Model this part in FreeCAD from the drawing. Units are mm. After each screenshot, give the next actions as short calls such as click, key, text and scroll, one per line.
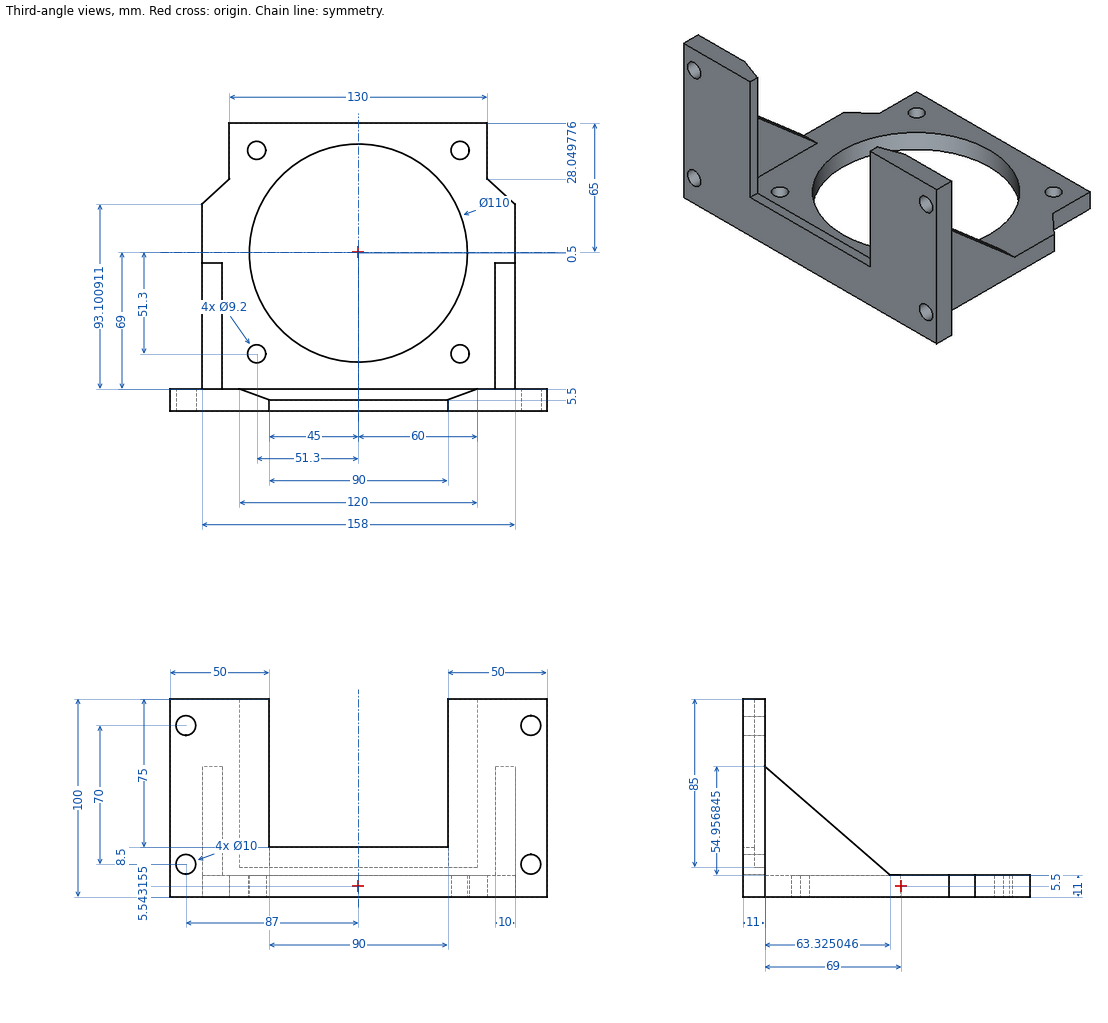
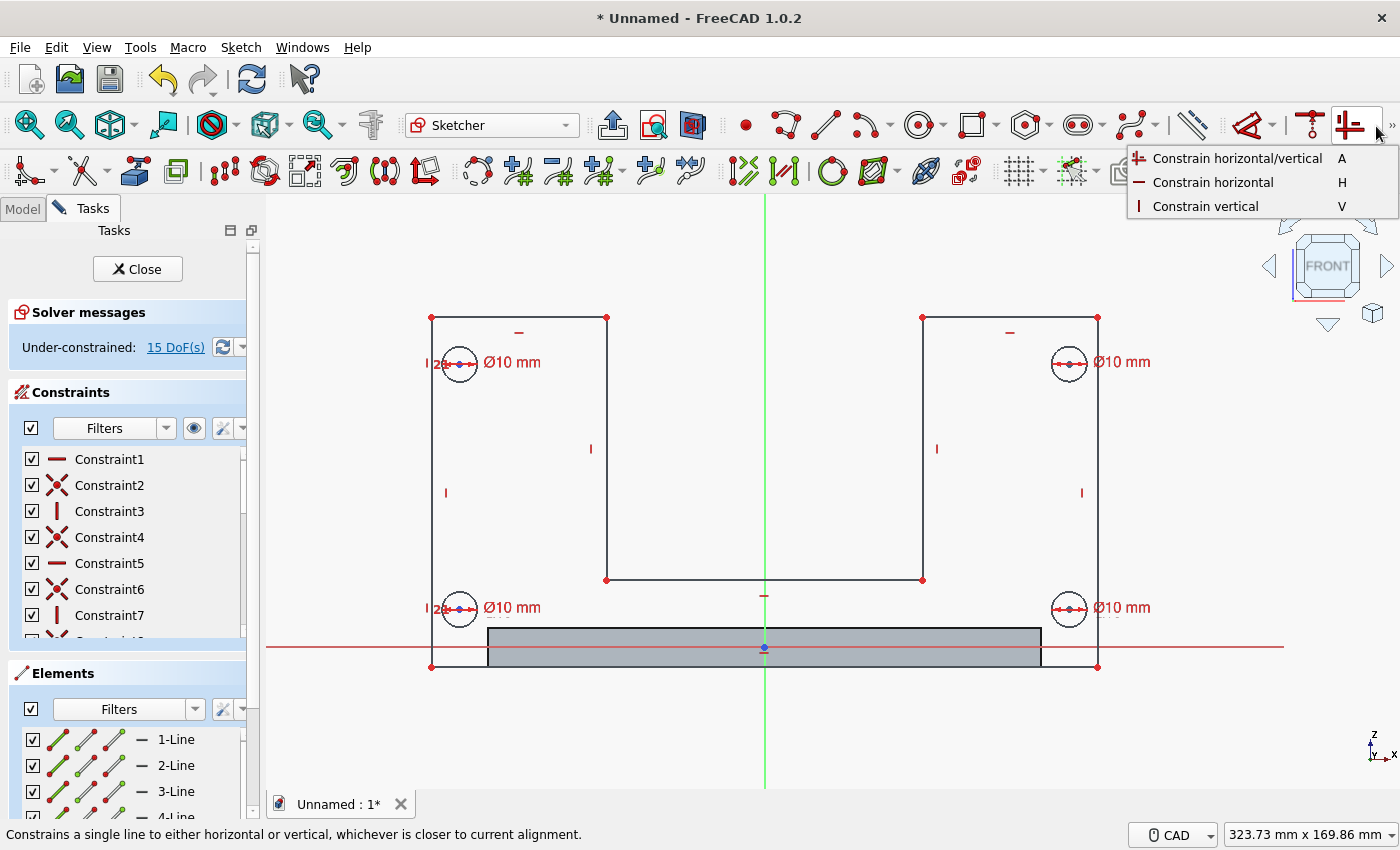
click(1263, 206)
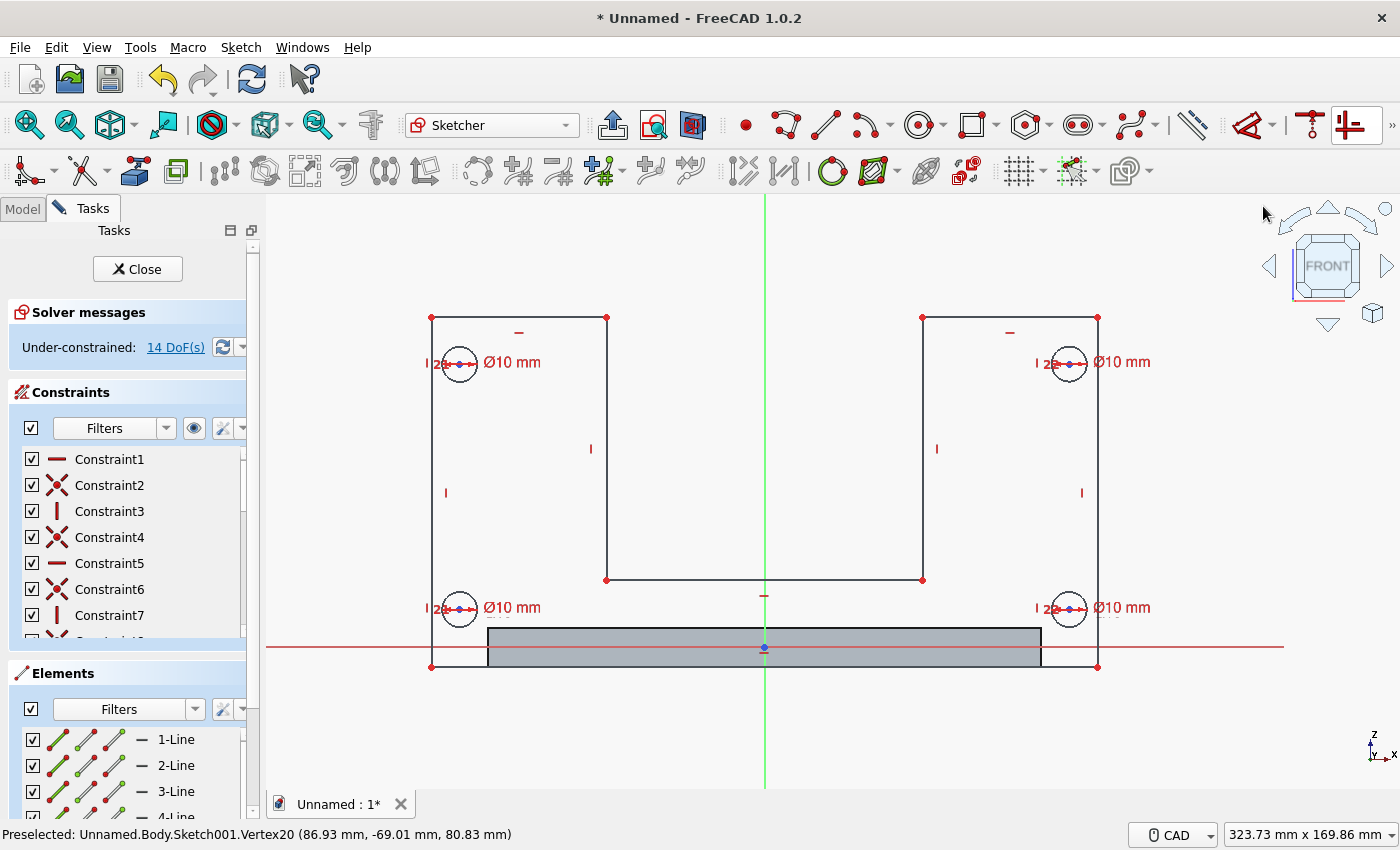
click(460, 610)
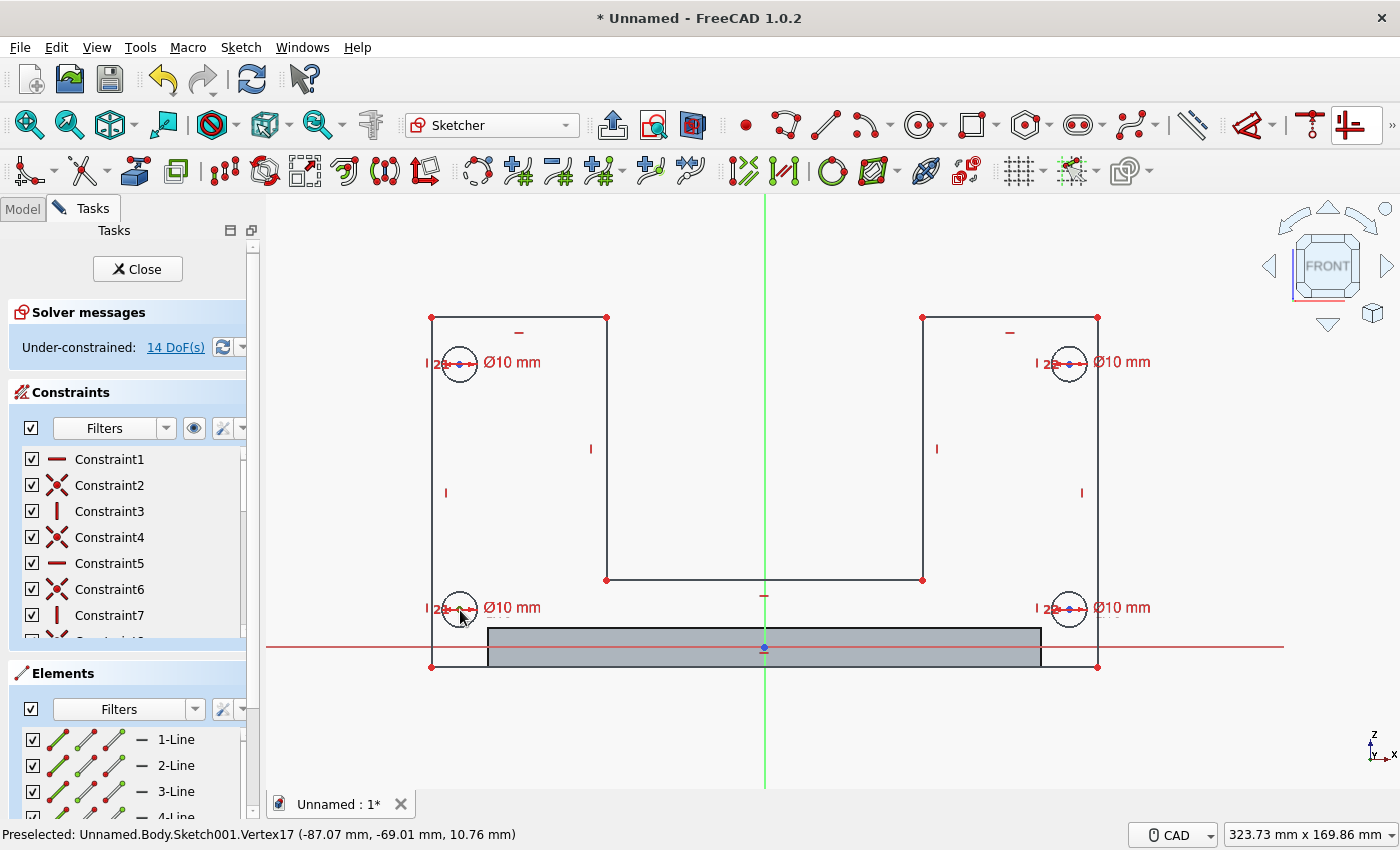
click(1069, 610)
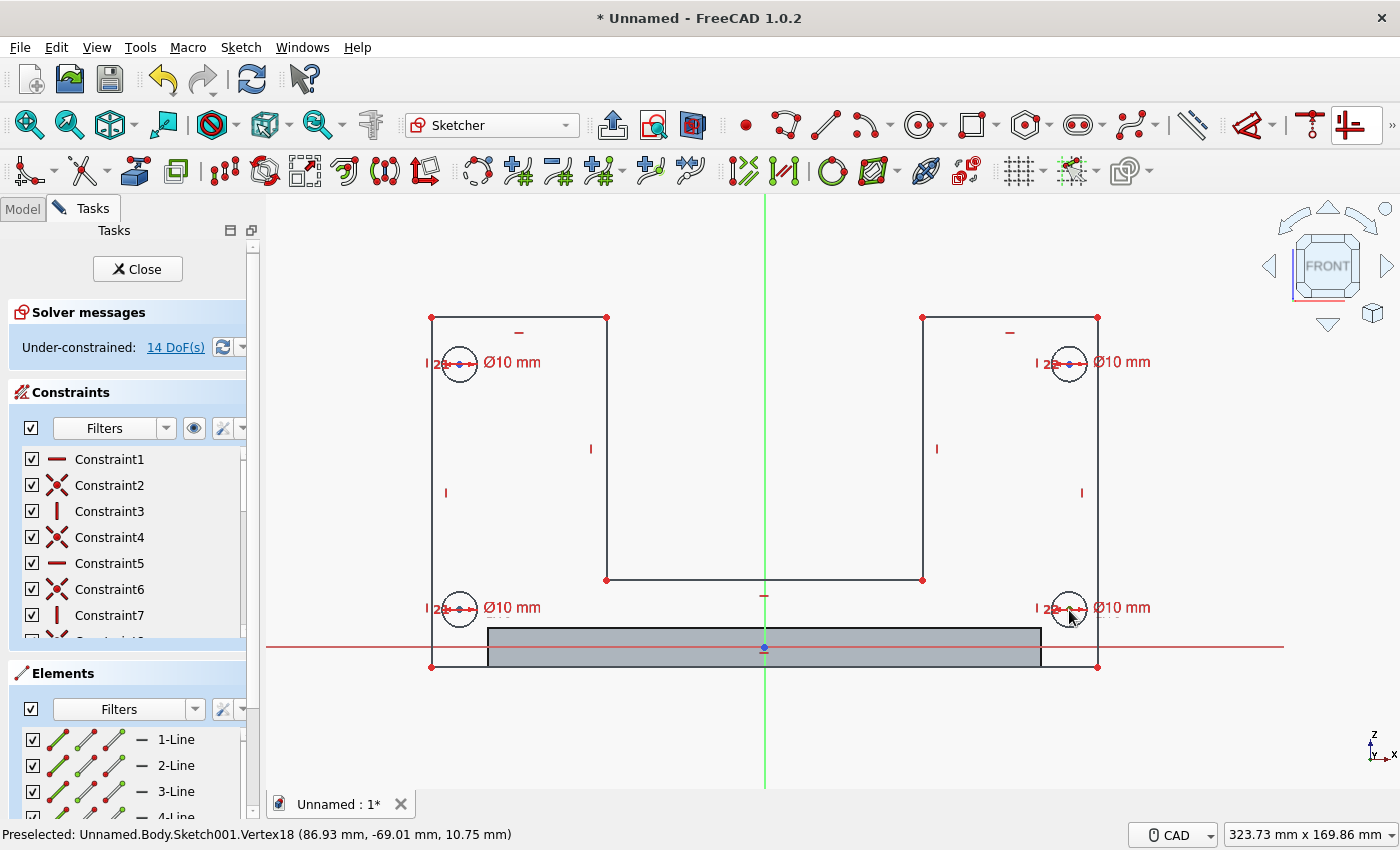
click(765, 722)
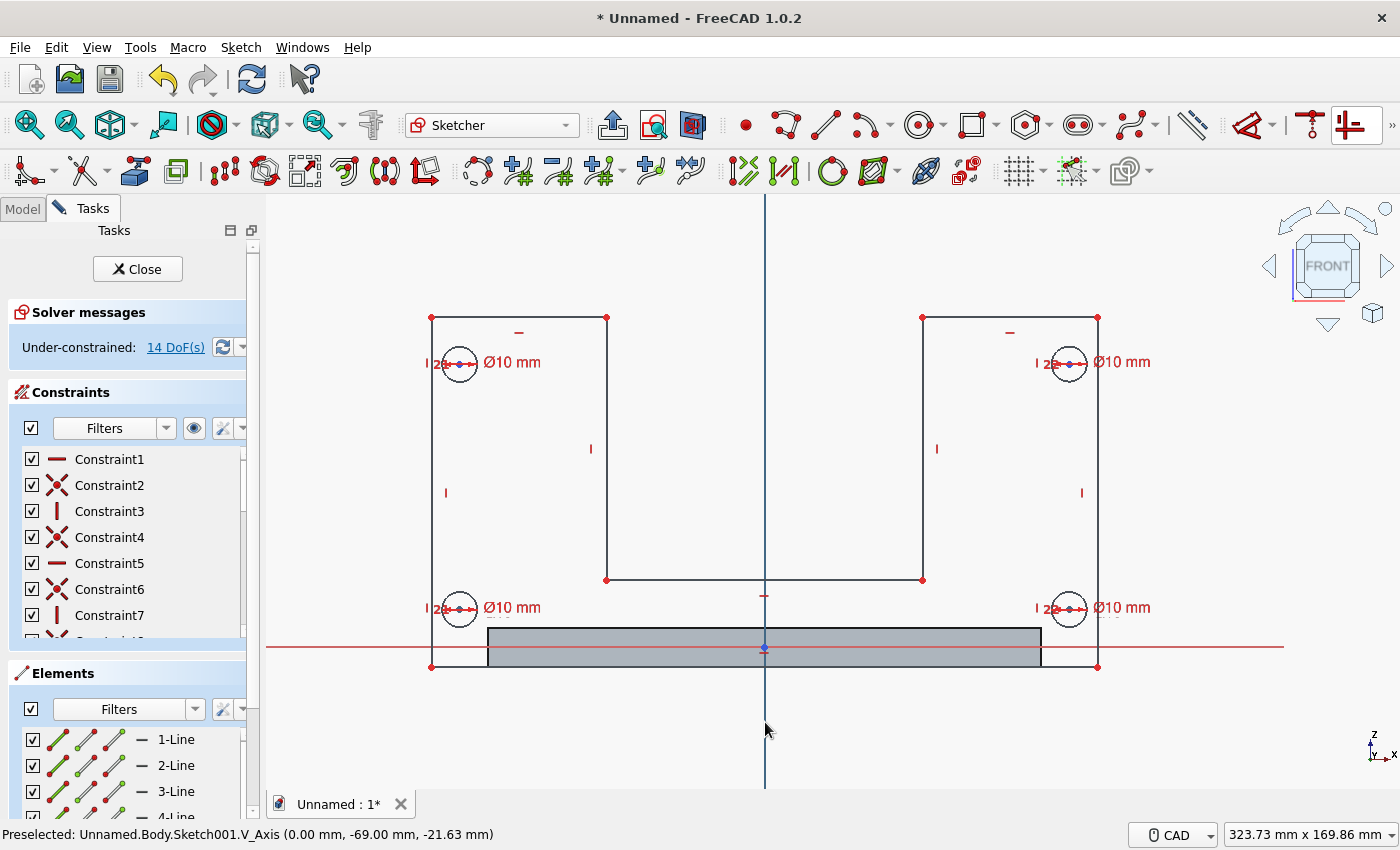
key(s)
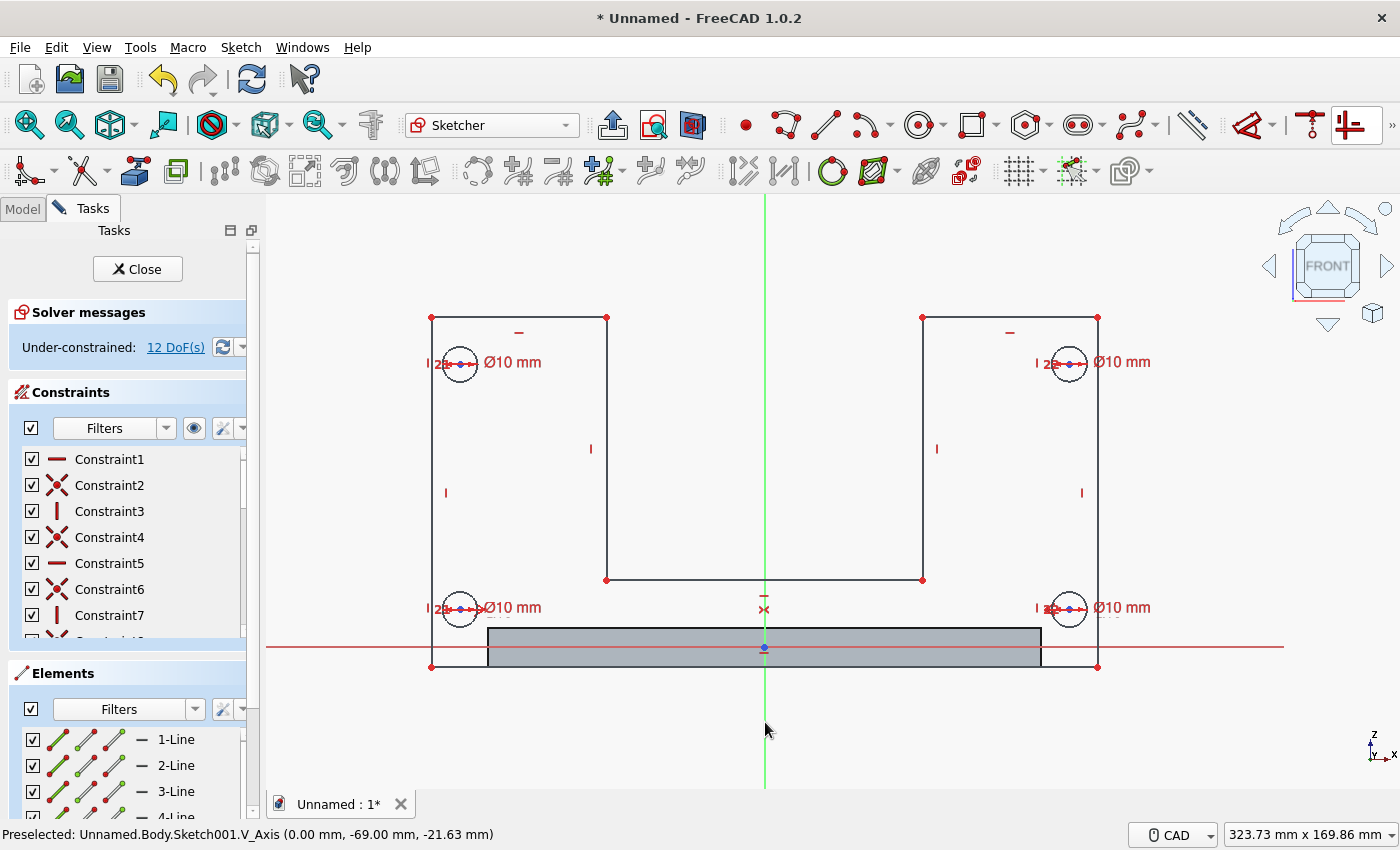
click(432, 317)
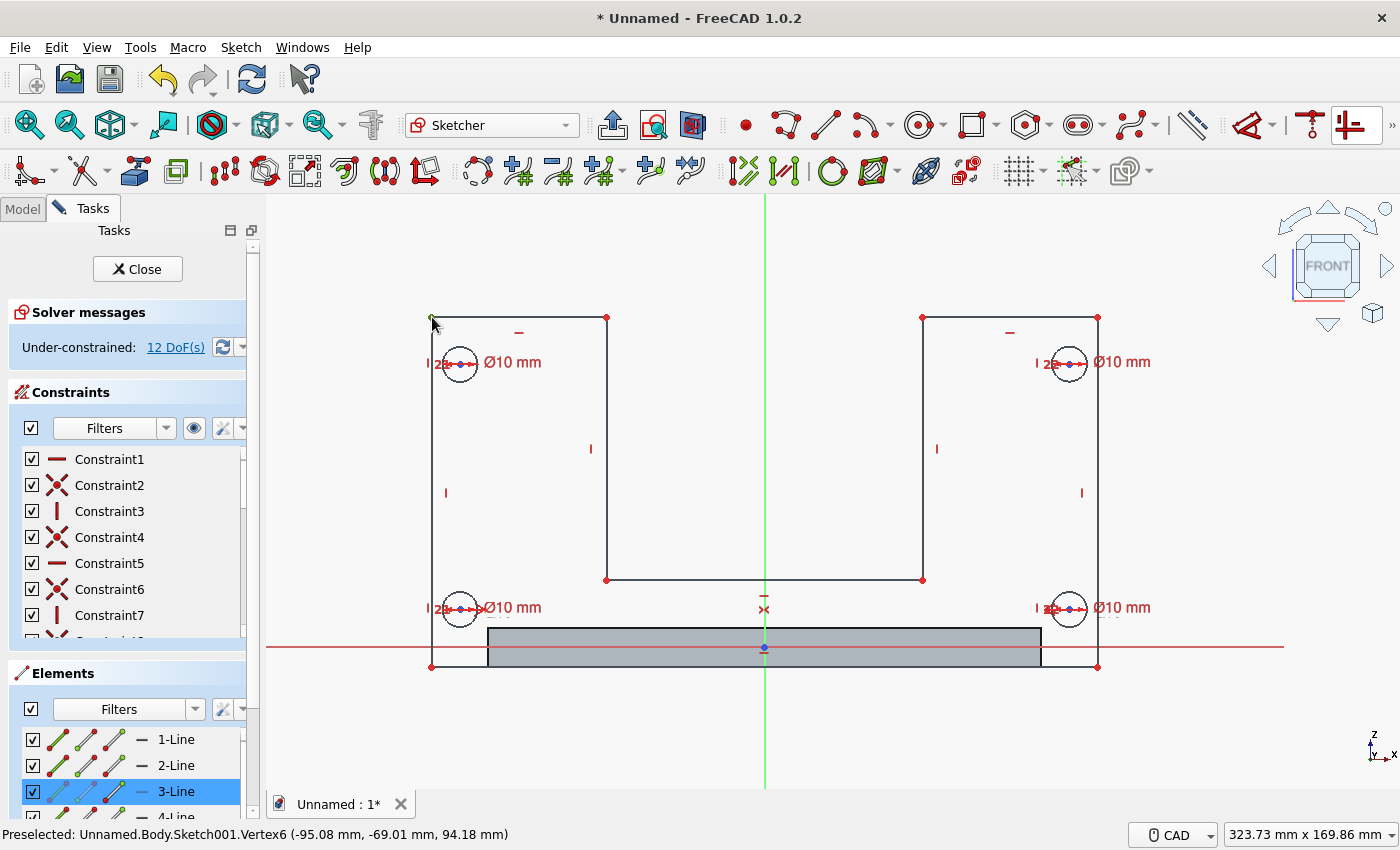
click(1098, 317)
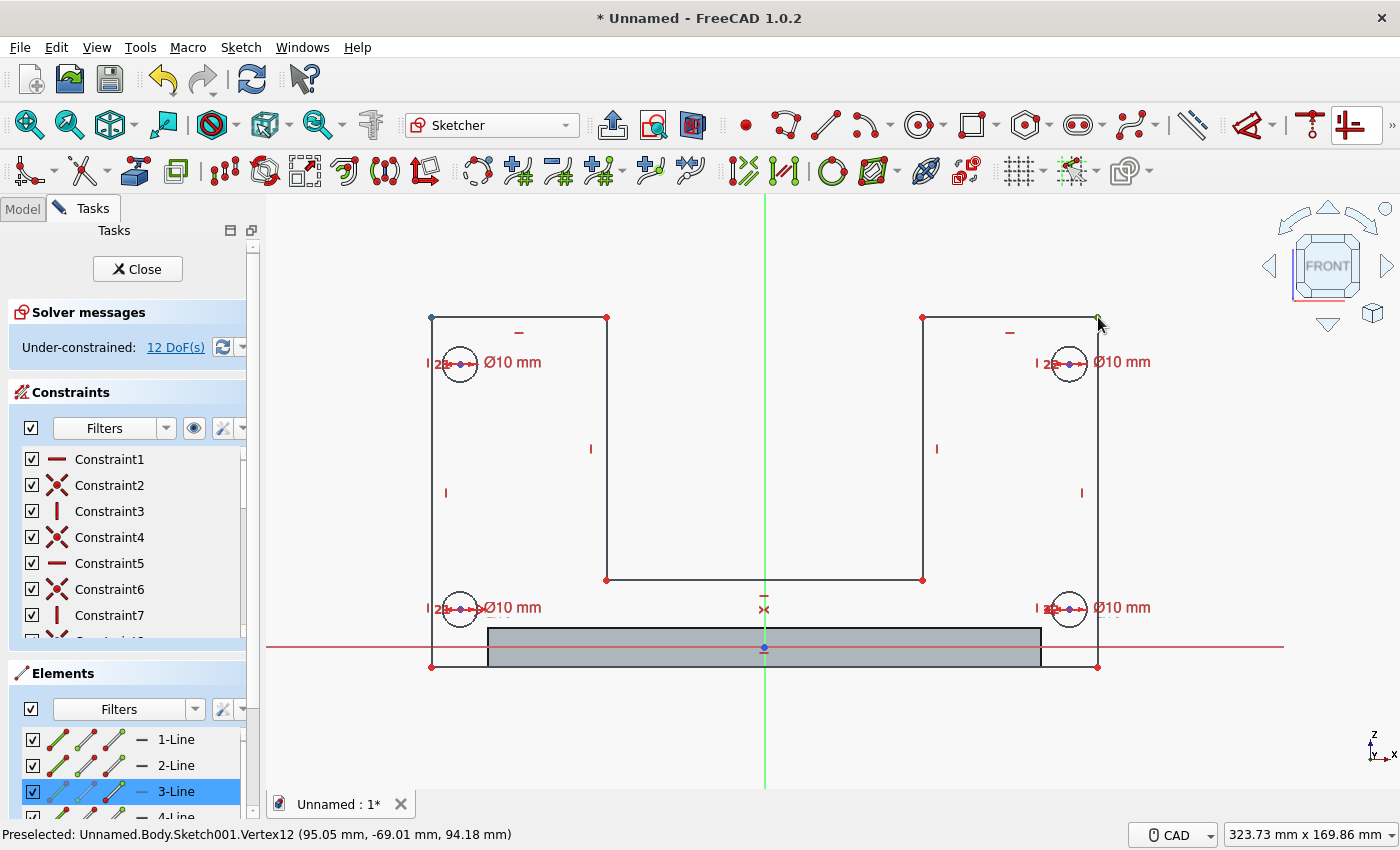
click(765, 722)